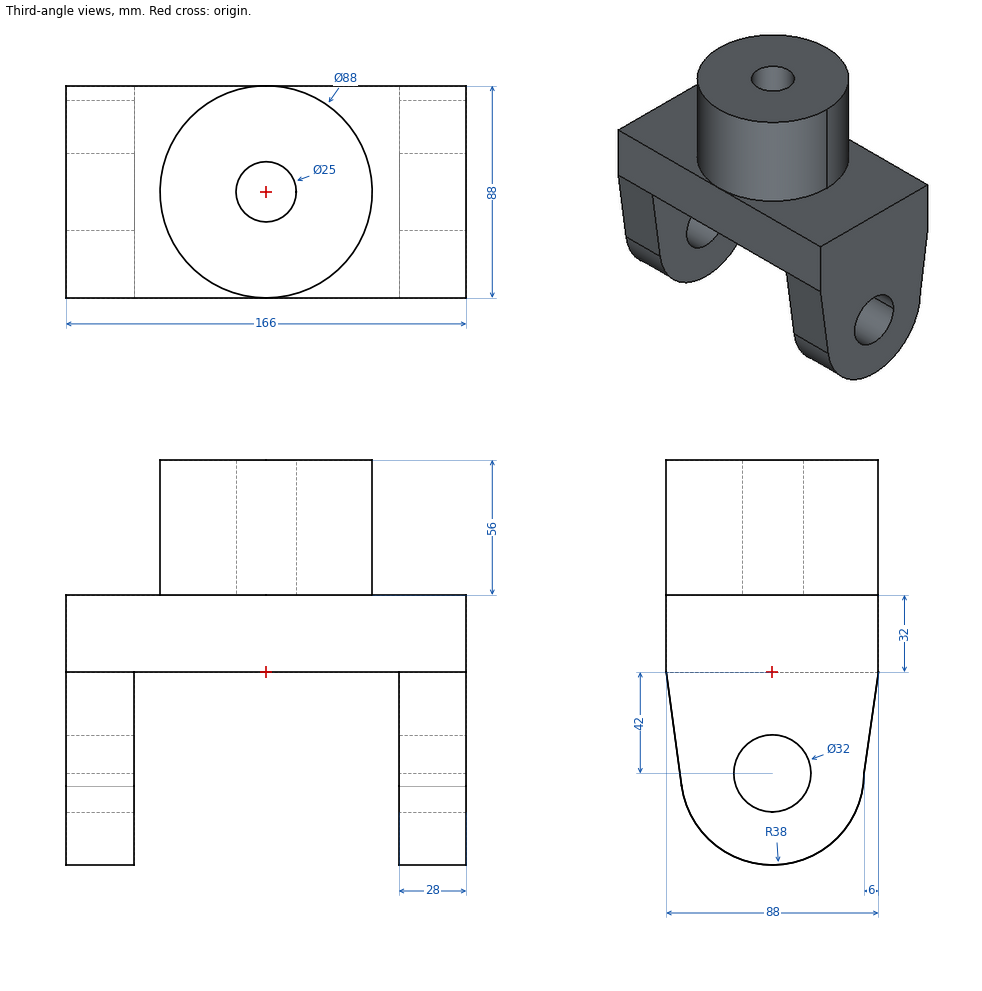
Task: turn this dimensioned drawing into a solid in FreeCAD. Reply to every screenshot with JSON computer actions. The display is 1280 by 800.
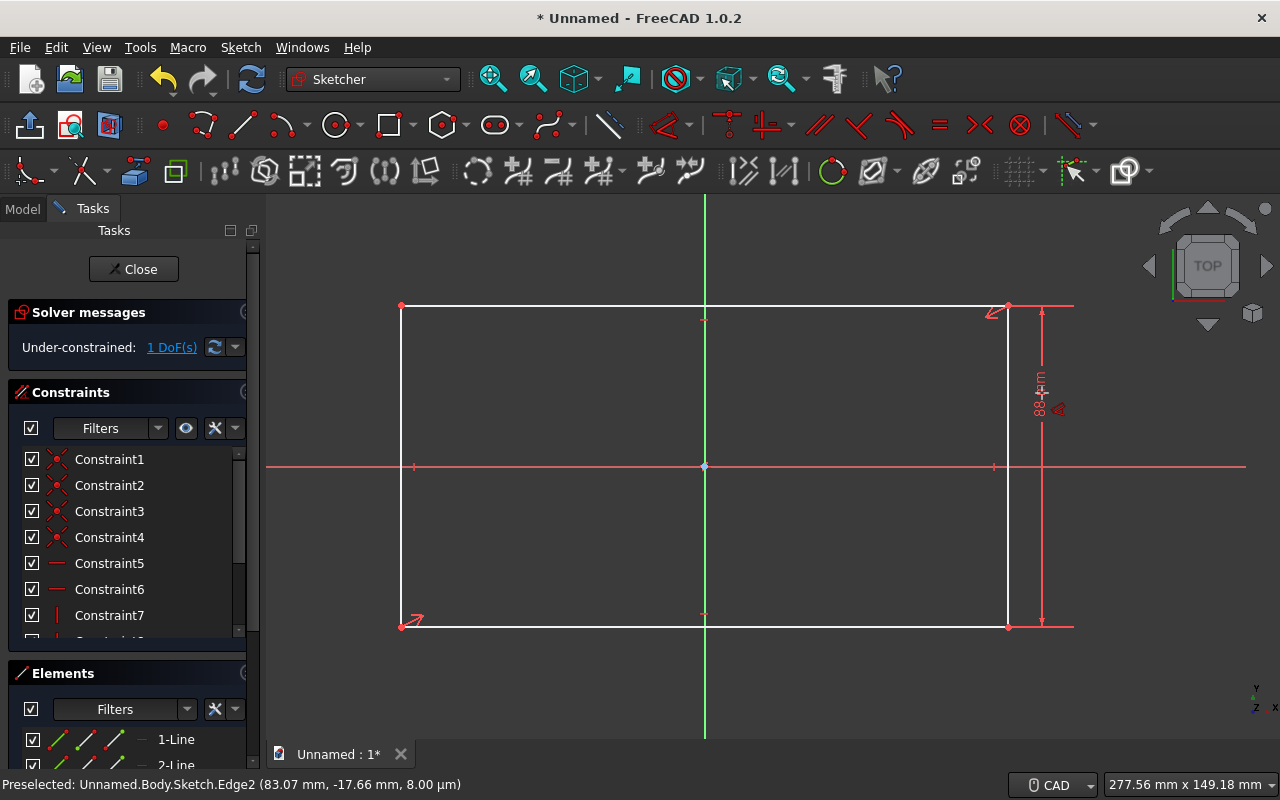
{"action": "left_click", "coordinate": [583, 627]}
{"action": "left_click", "coordinate": [565, 661]}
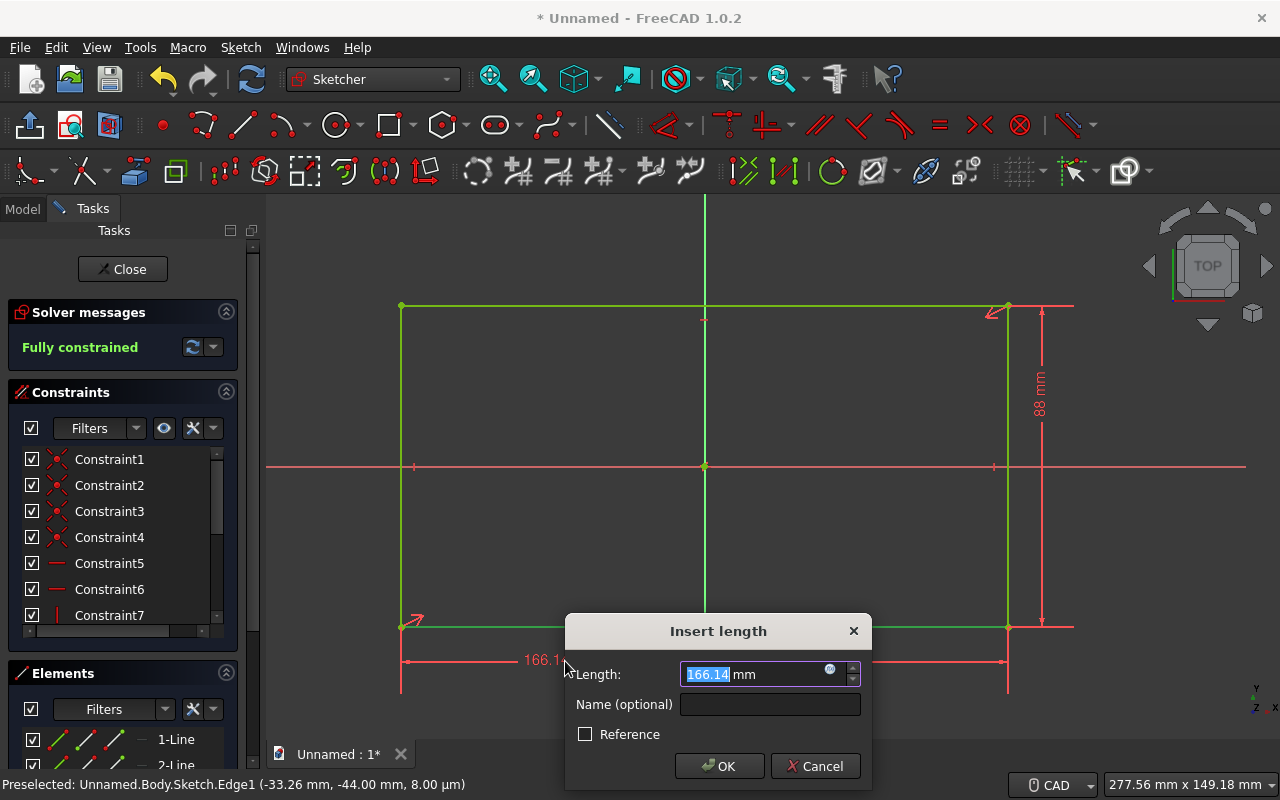
{"action": "type", "text": "166"}
{"action": "key", "text": "Return"}
{"action": "key", "text": "Escape"}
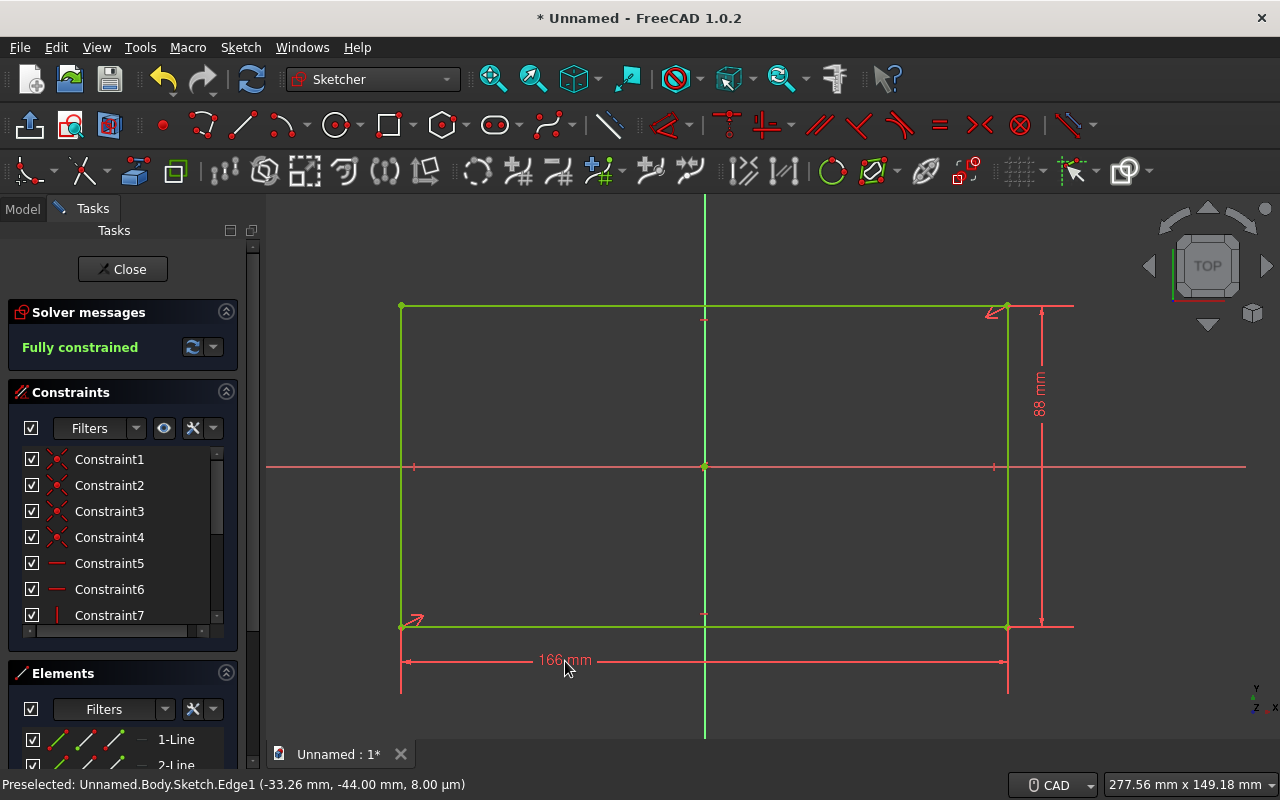
{"action": "left_click", "coordinate": [123, 269]}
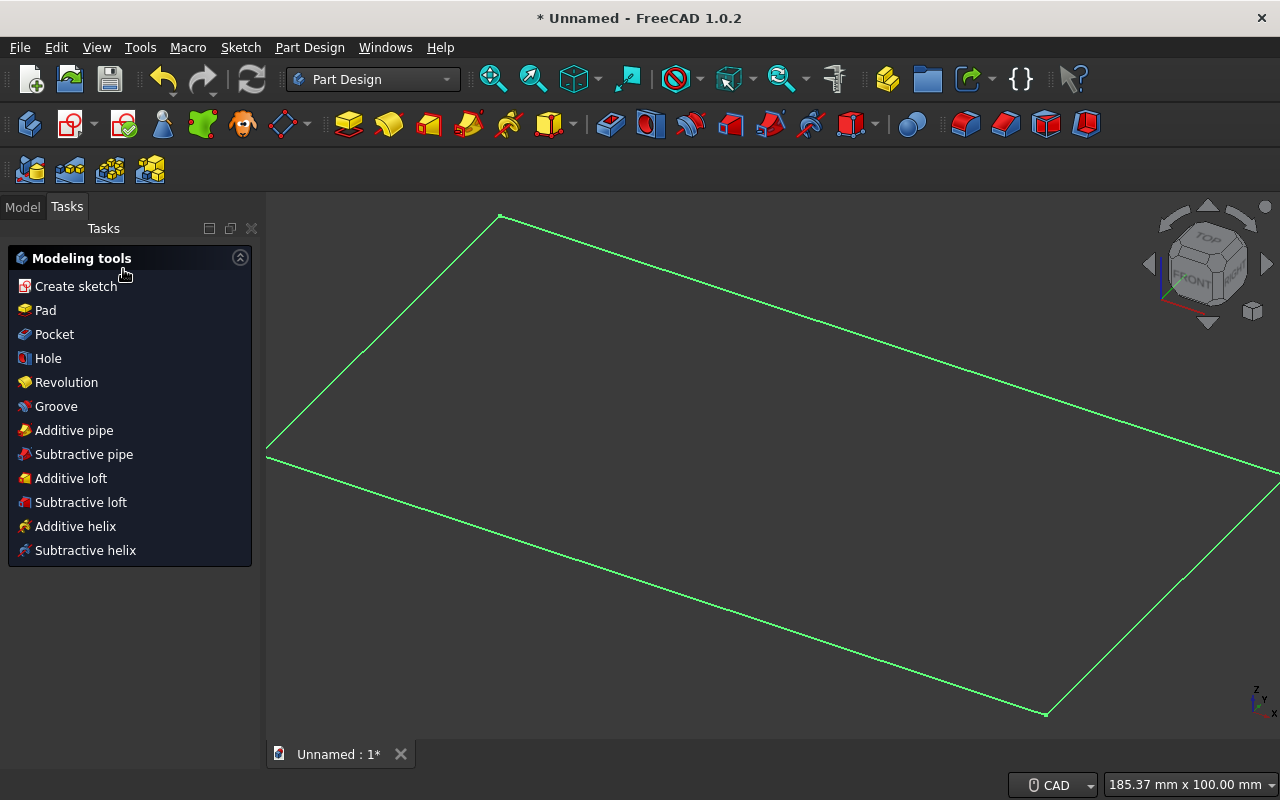
{"action": "left_click", "coordinate": [350, 124]}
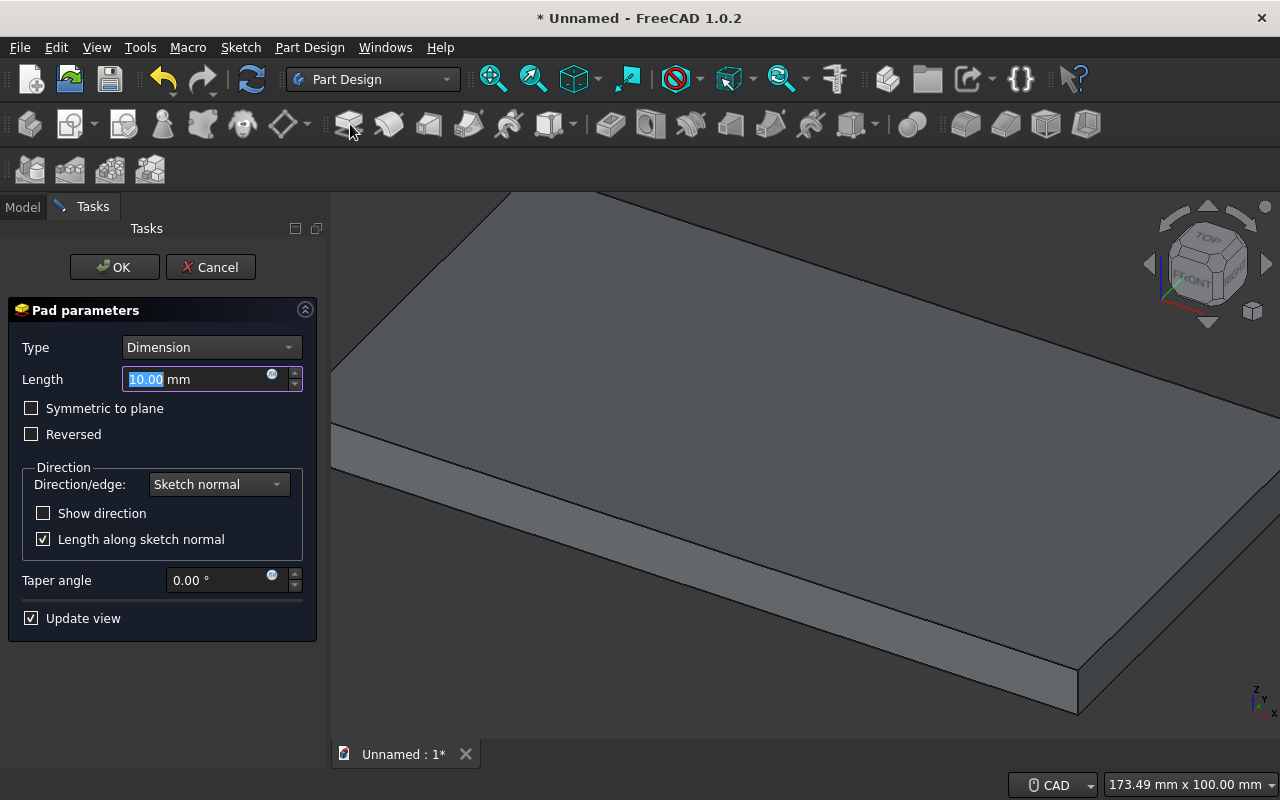
{"action": "type", "text": "32"}
{"action": "key", "text": "Tab"}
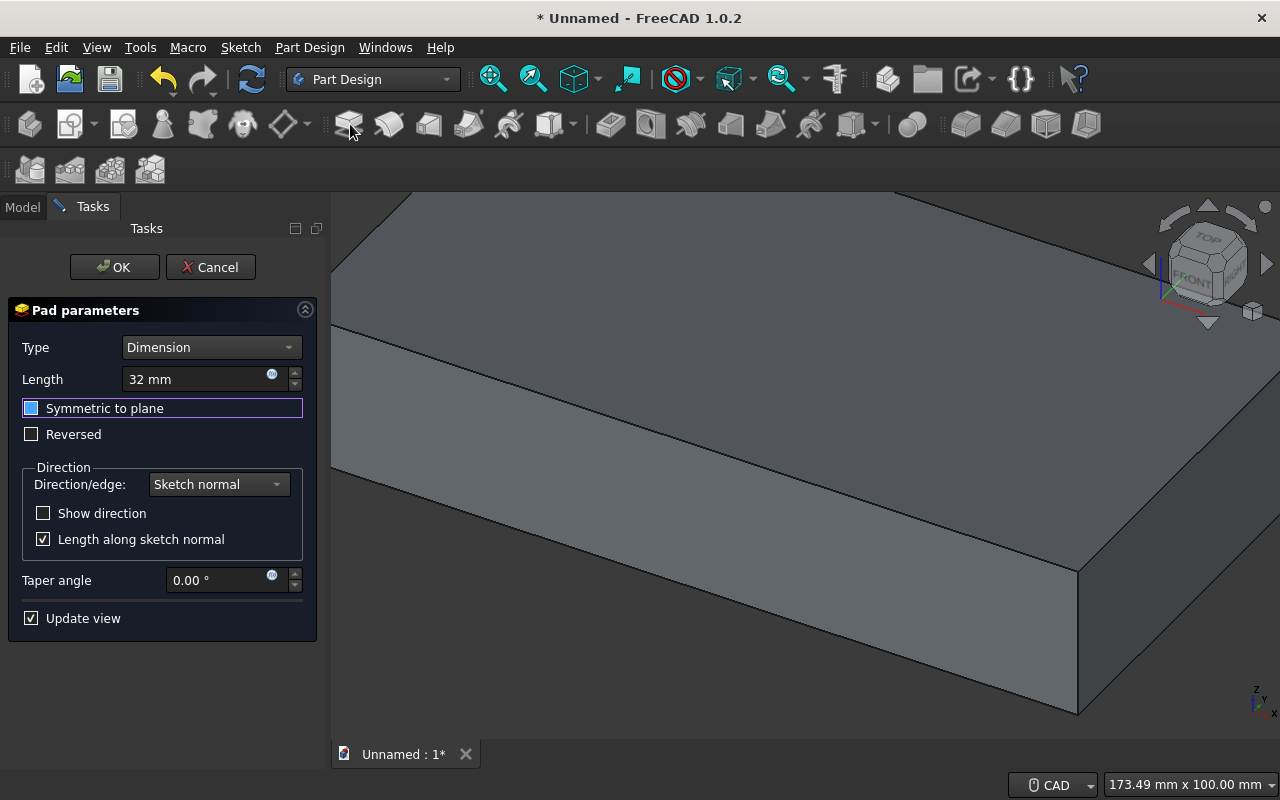
{"action": "left_click", "coordinate": [115, 267]}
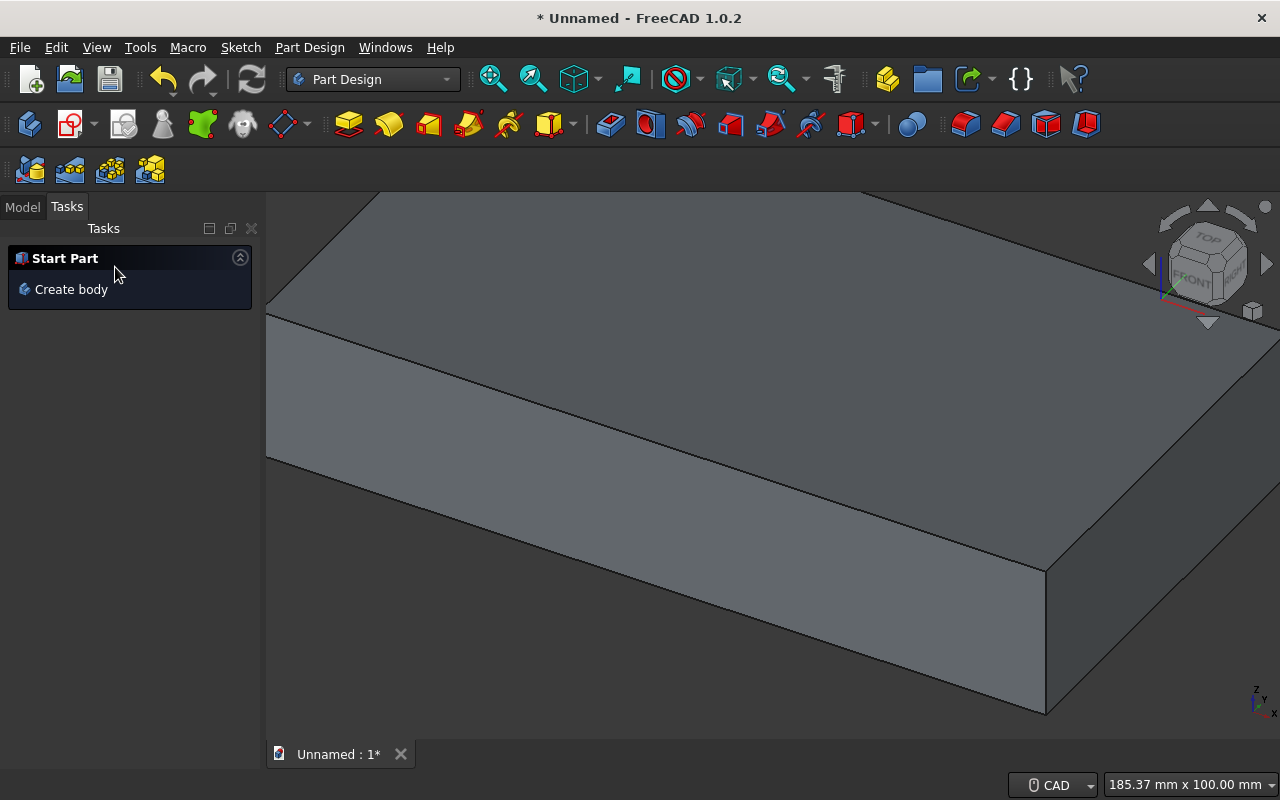
{"action": "left_click", "coordinate": [494, 80]}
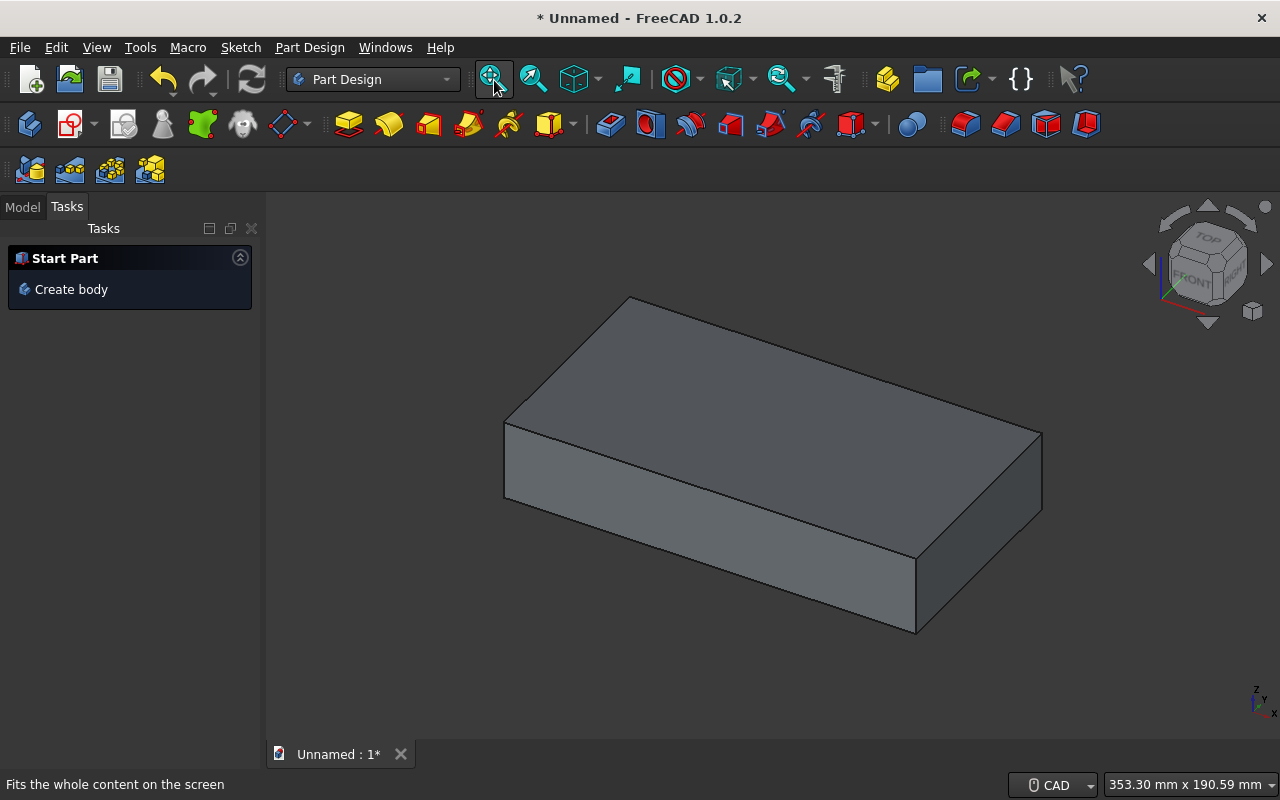
{"action": "left_click", "coordinate": [832, 446]}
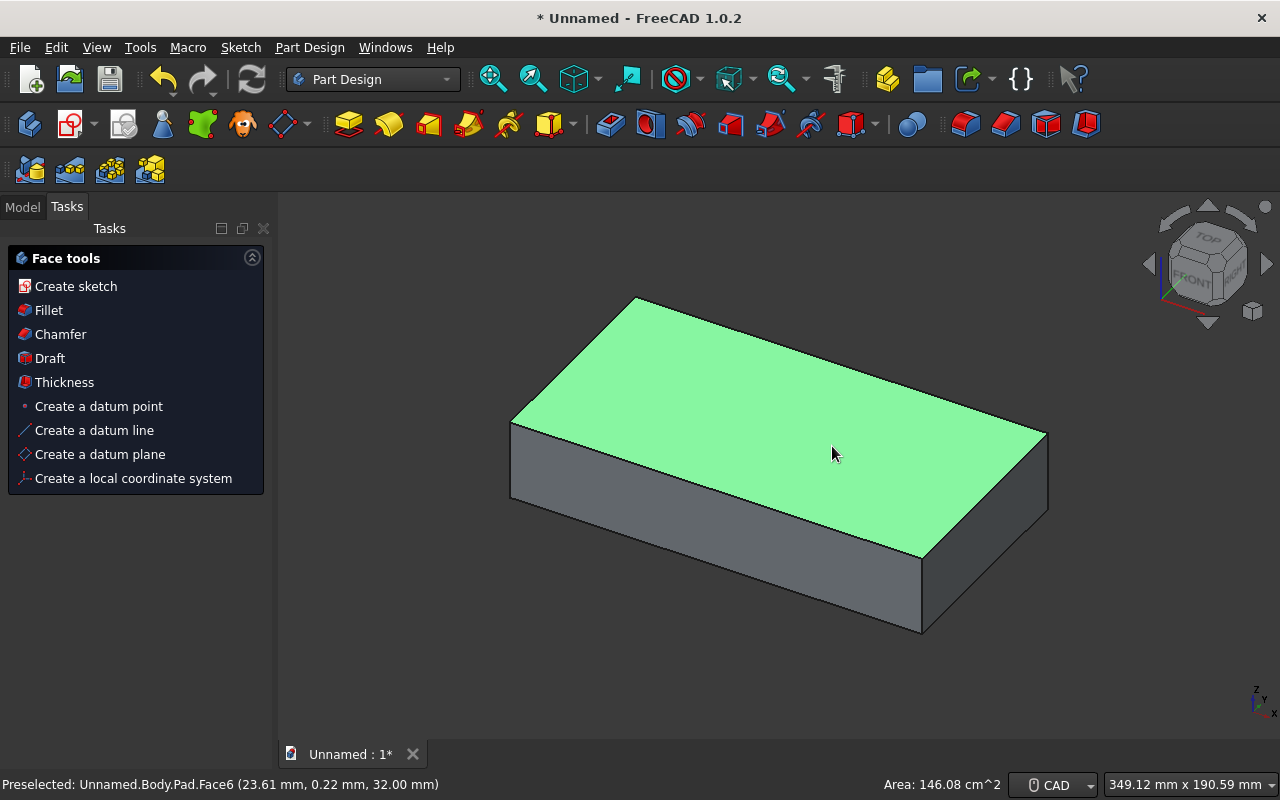
{"action": "left_click", "coordinate": [70, 124]}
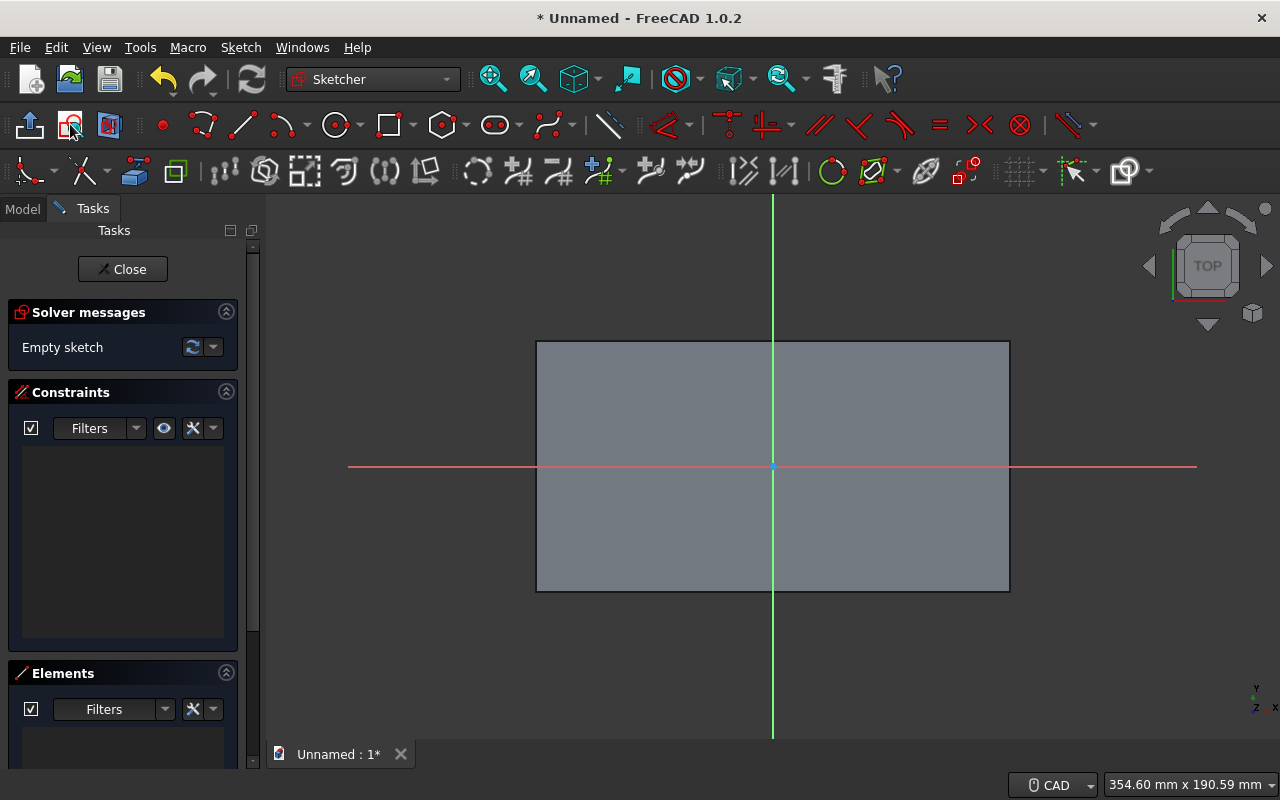
{"action": "scroll", "coordinate": [912, 467], "scroll_direction": "up", "scroll_amount": 2}